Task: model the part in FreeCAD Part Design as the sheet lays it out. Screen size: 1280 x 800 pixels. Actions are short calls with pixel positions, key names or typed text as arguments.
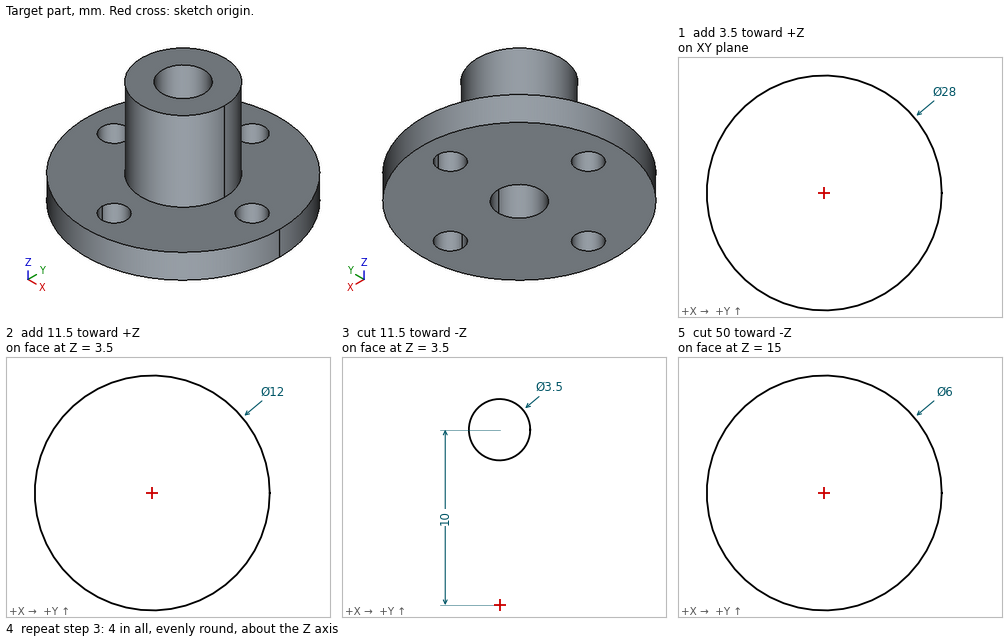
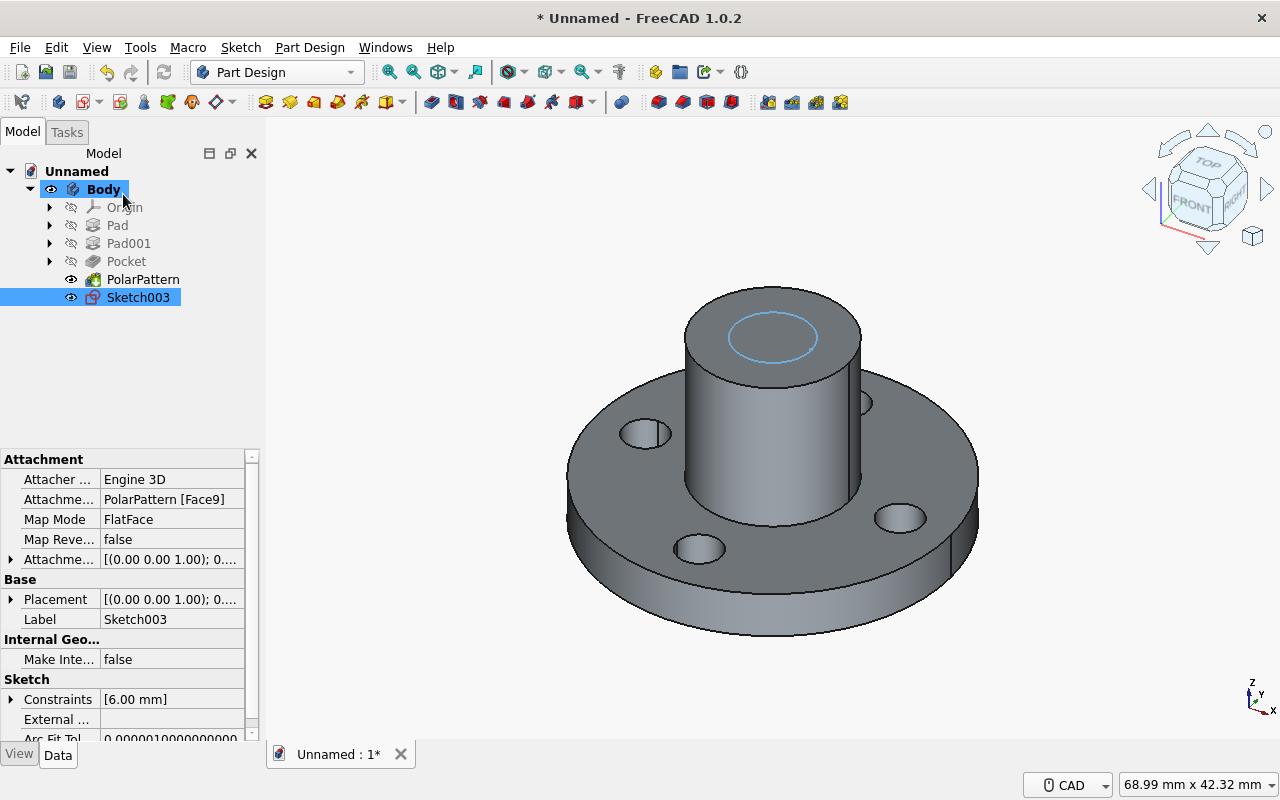
click(432, 102)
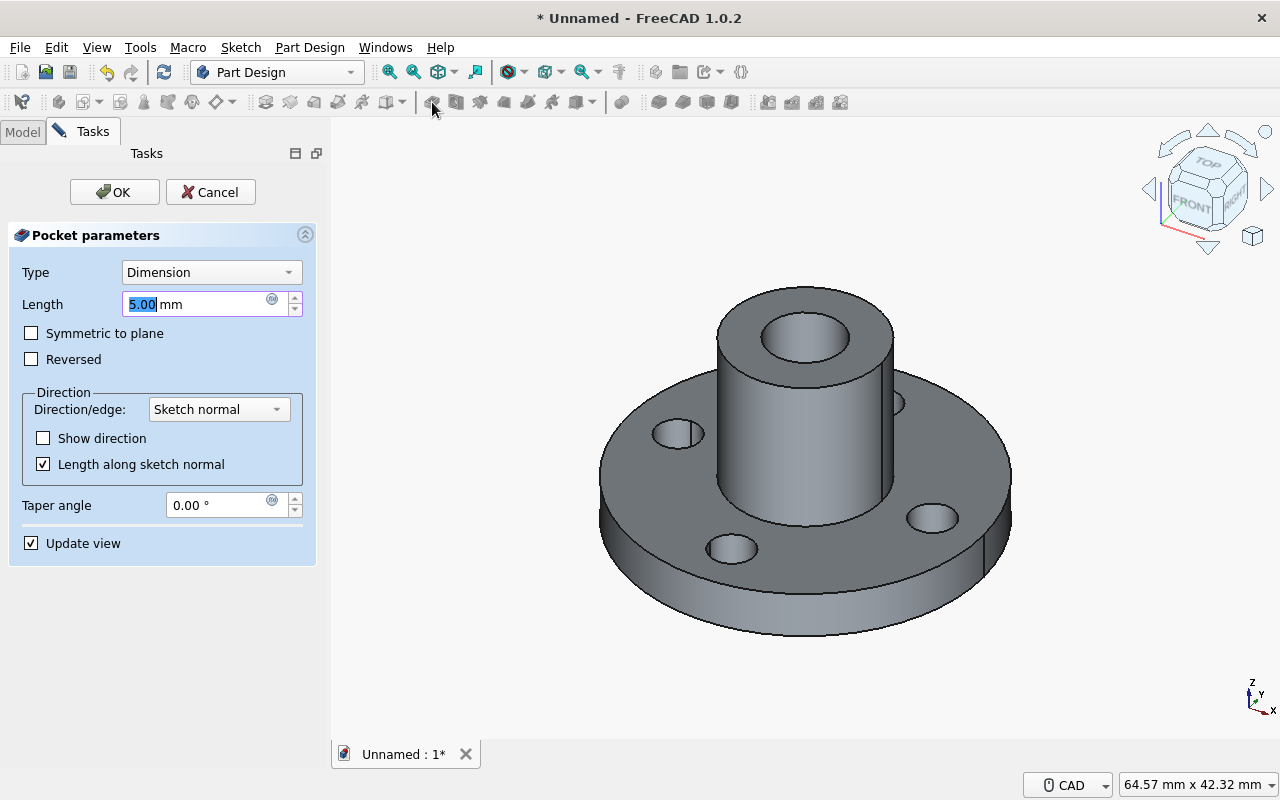
text(50)
key(Tab)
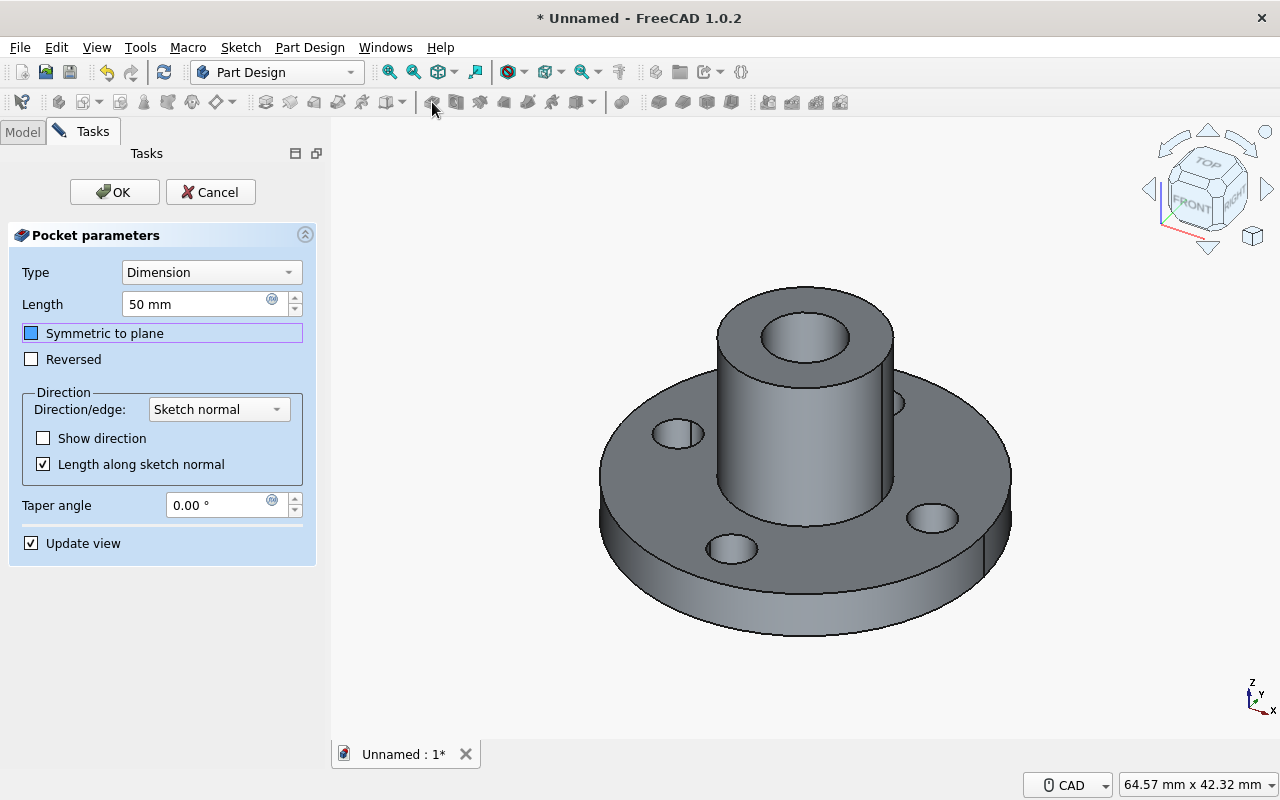
click(115, 192)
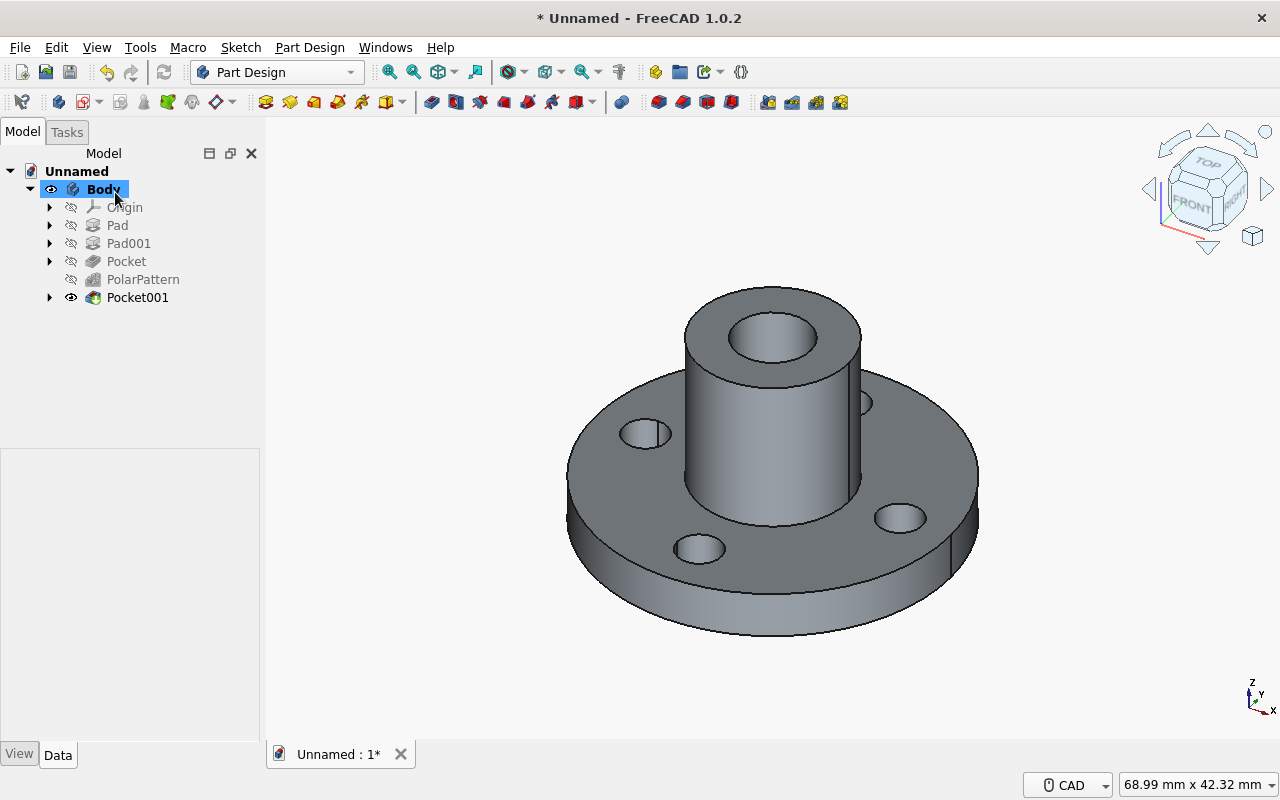
key(0)